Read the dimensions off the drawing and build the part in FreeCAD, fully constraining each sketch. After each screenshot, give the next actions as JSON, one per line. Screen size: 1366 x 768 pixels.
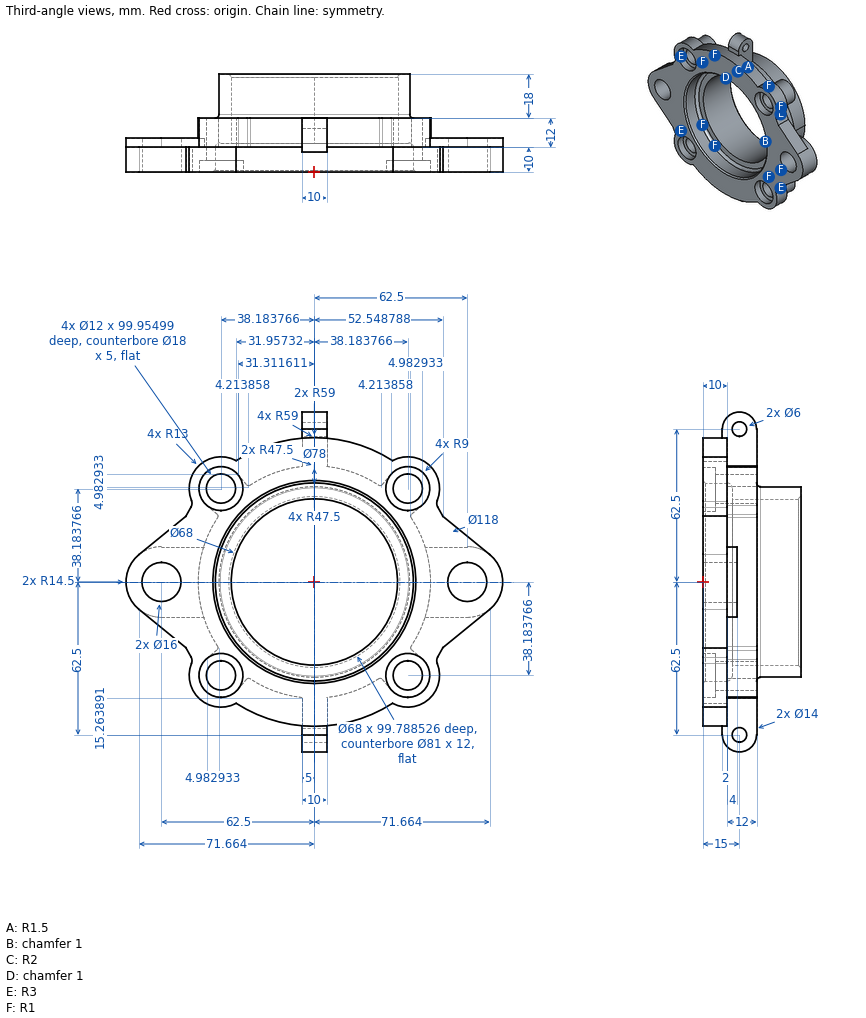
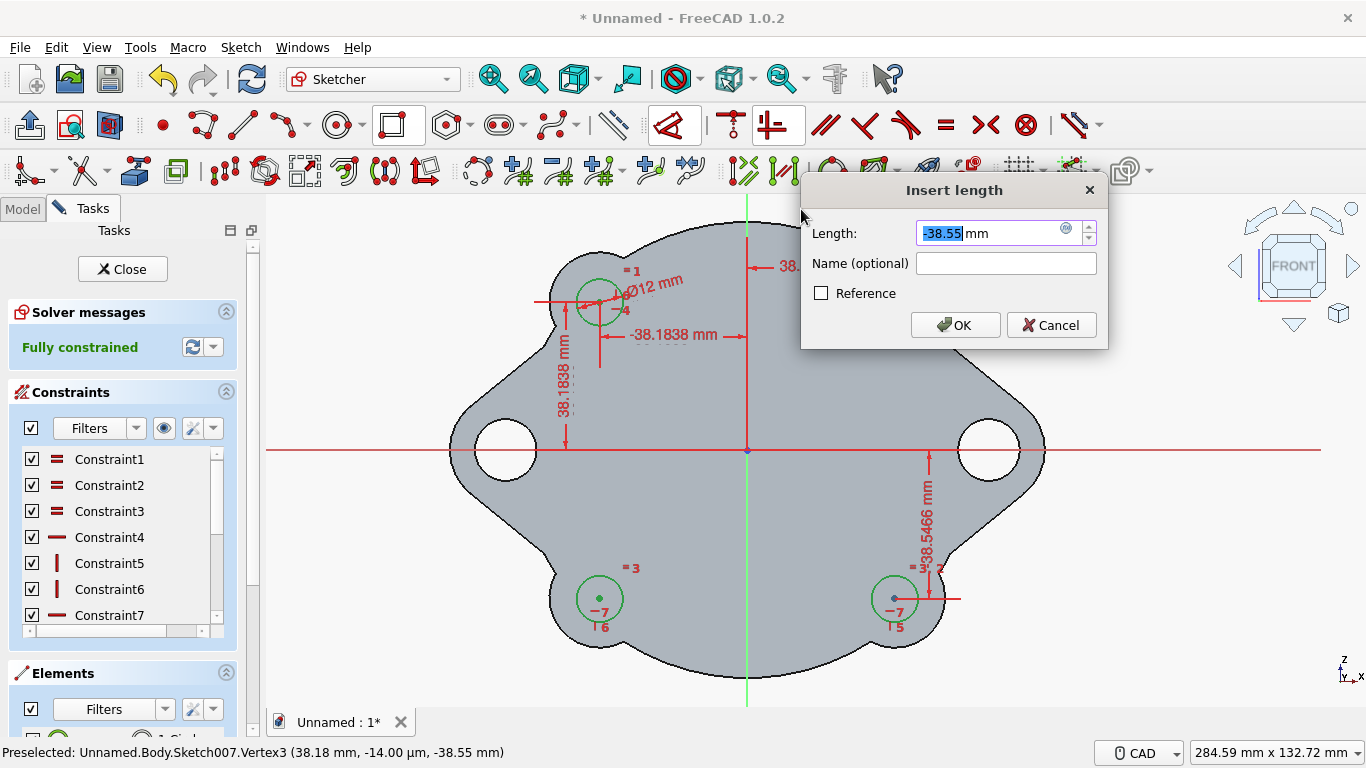
{"action": "type", "text": "-38.183766"}
{"action": "key", "text": "Return"}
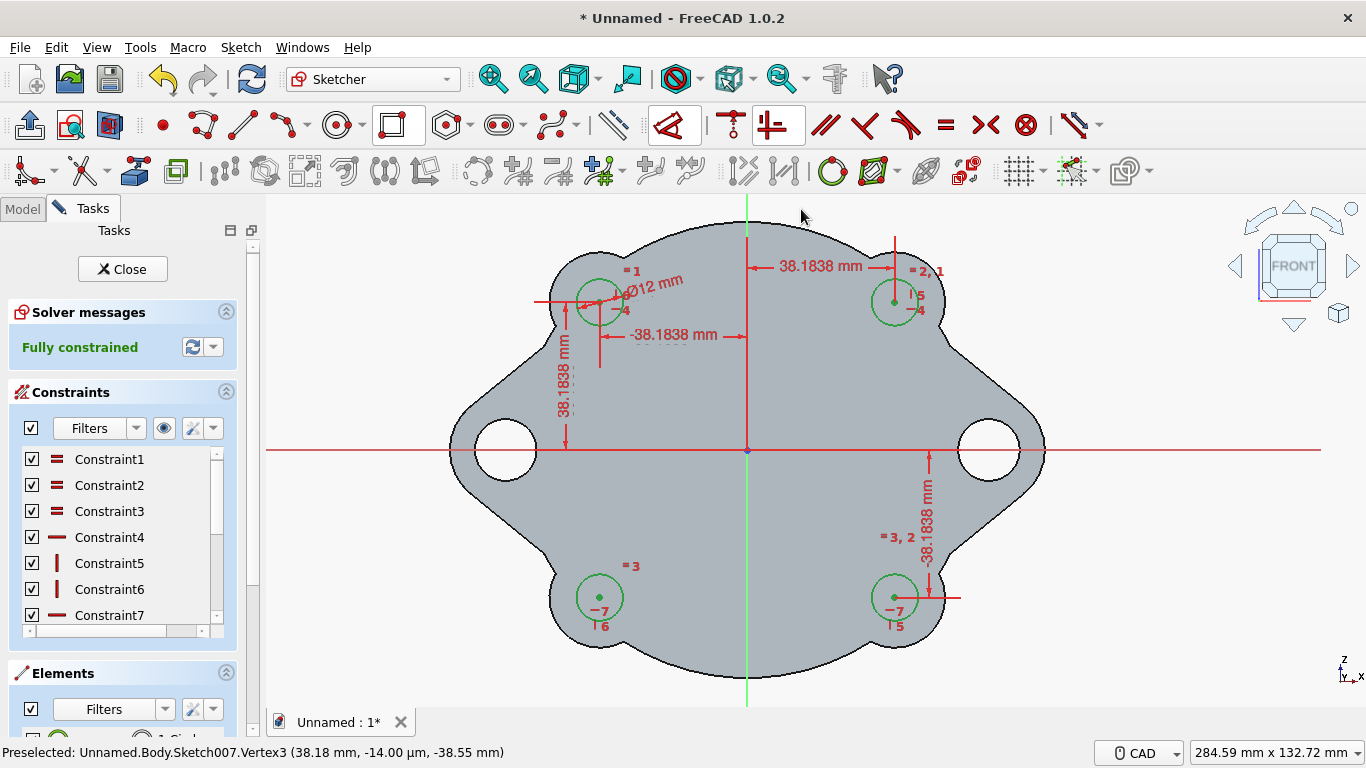
{"action": "left_click", "coordinate": [123, 269]}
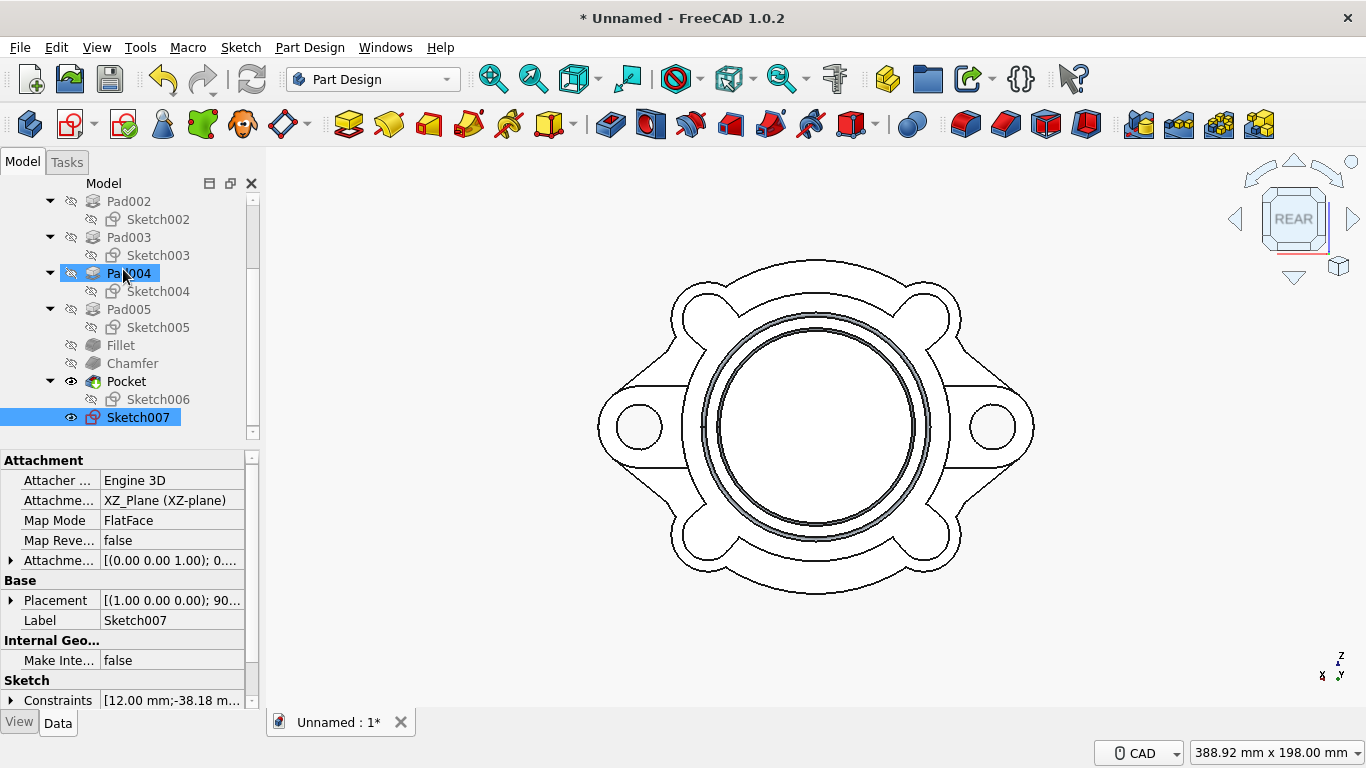
{"action": "left_click", "coordinate": [652, 124]}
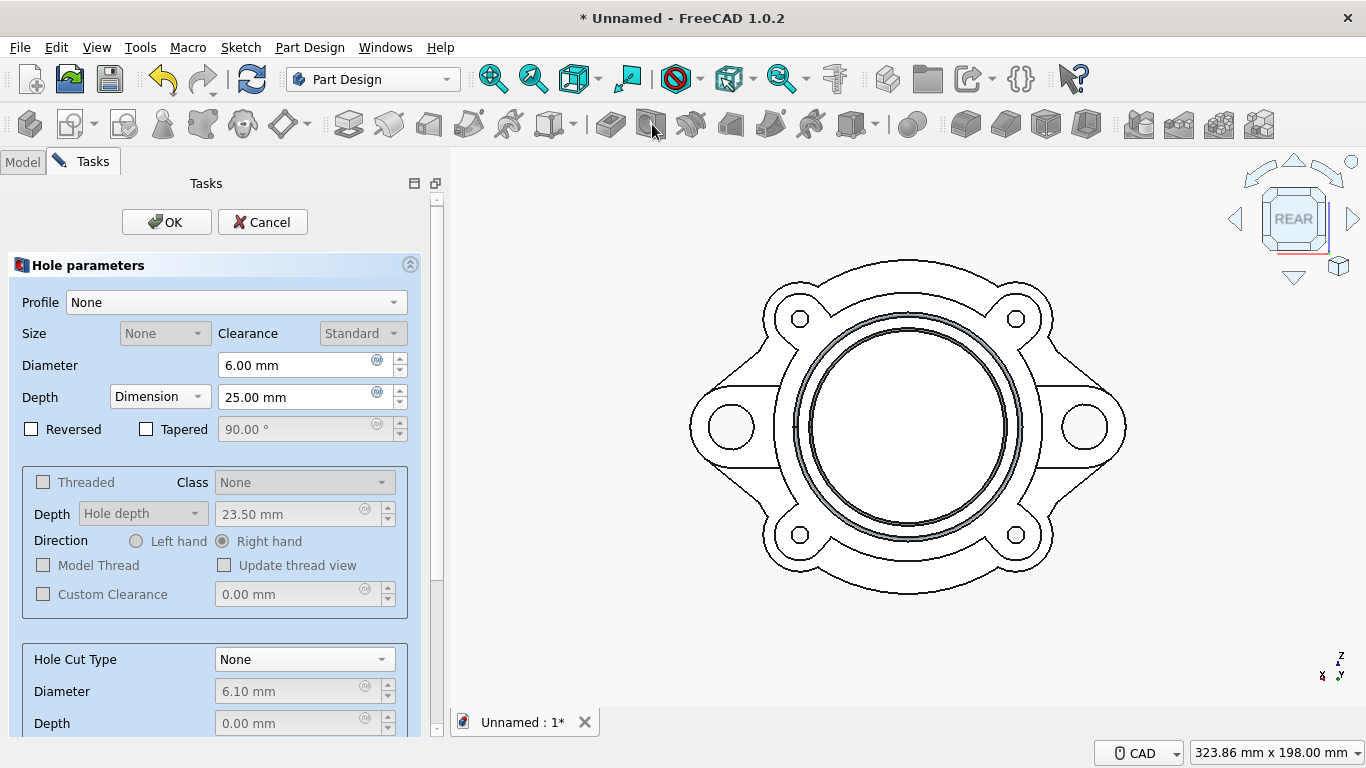
{"action": "triple_click", "coordinate": [305, 365]}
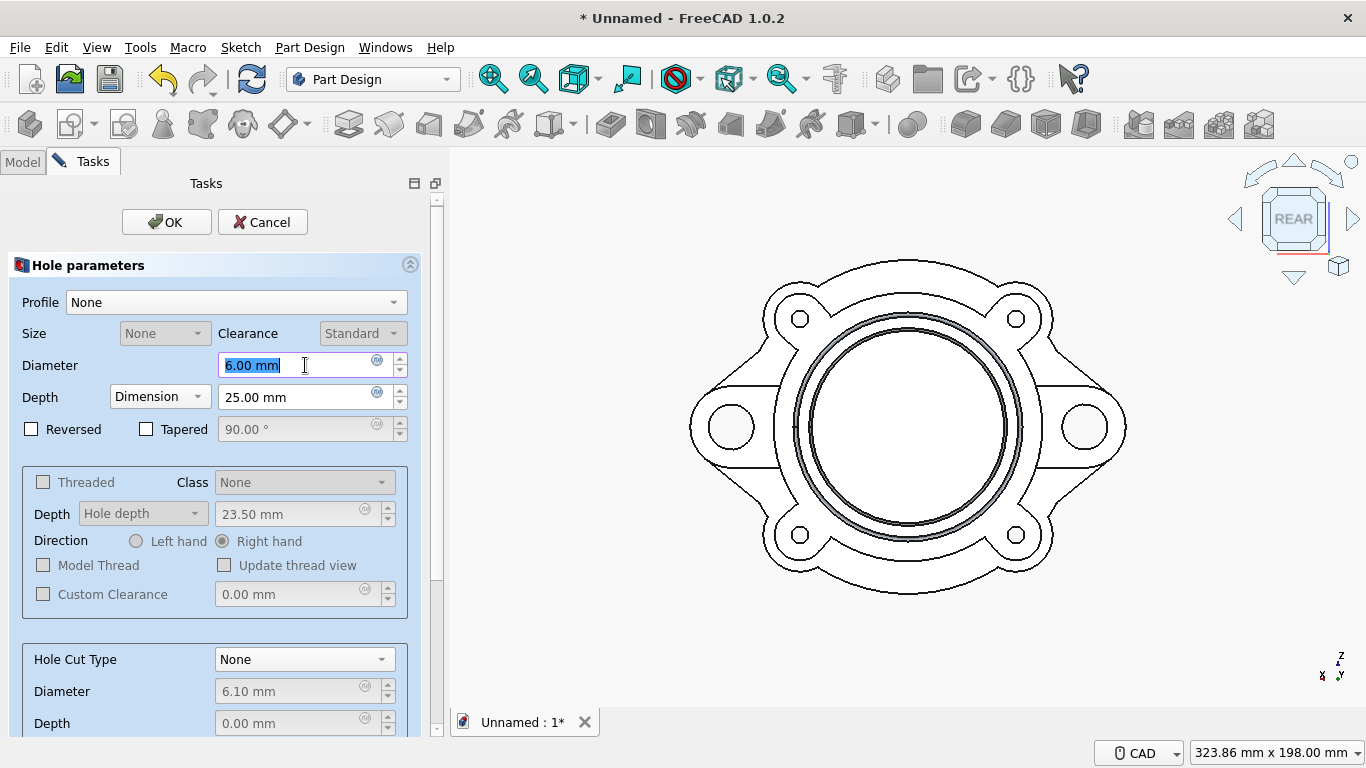
{"action": "type", "text": "12"}
{"action": "key", "text": "Tab"}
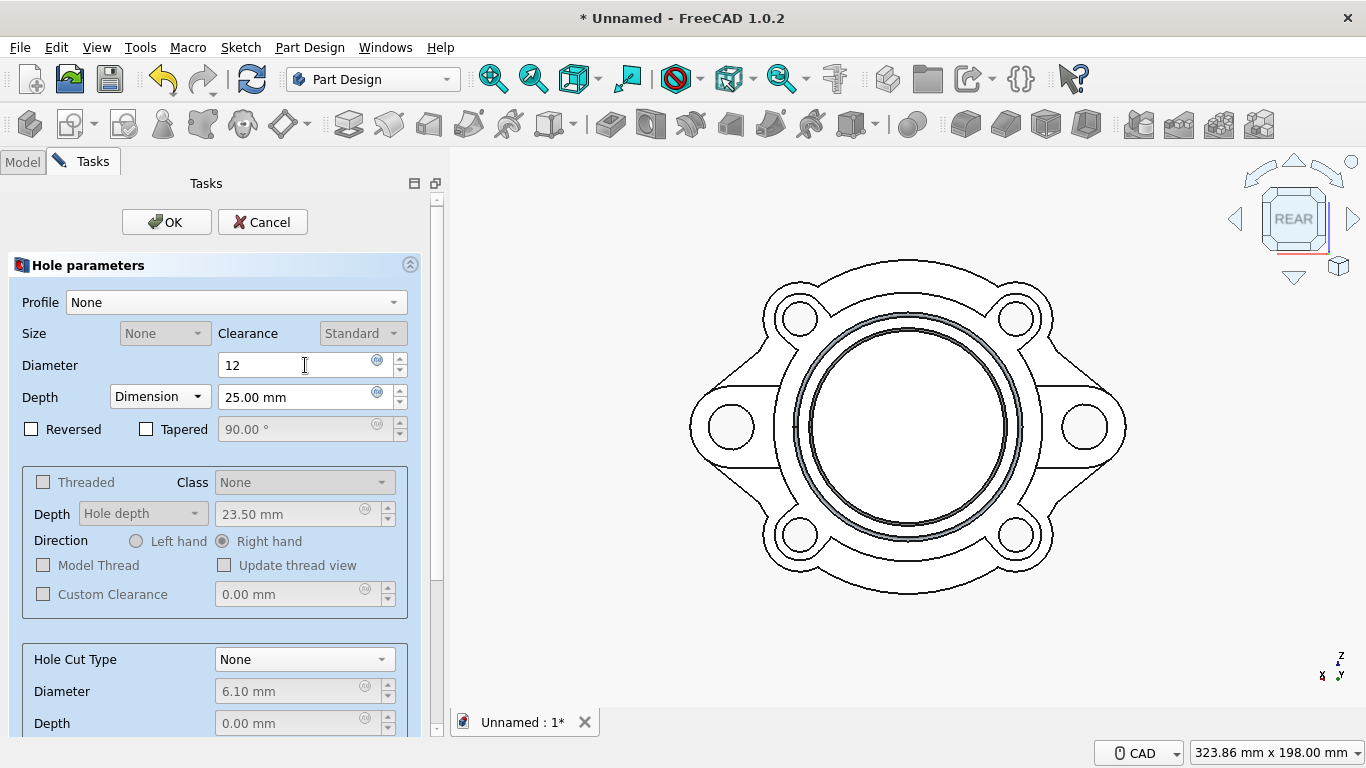
{"action": "triple_click", "coordinate": [305, 397]}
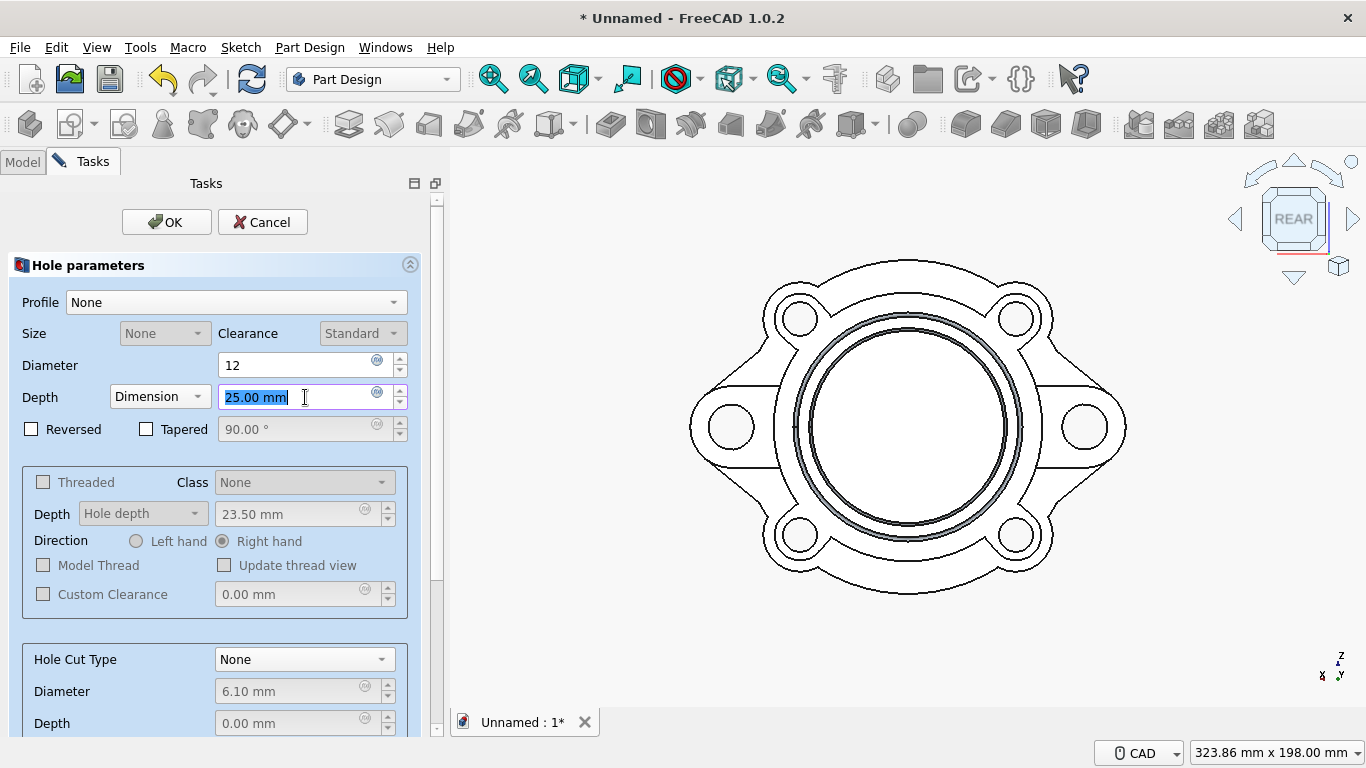
{"action": "type", "text": "99.95499"}
{"action": "key", "text": "Tab"}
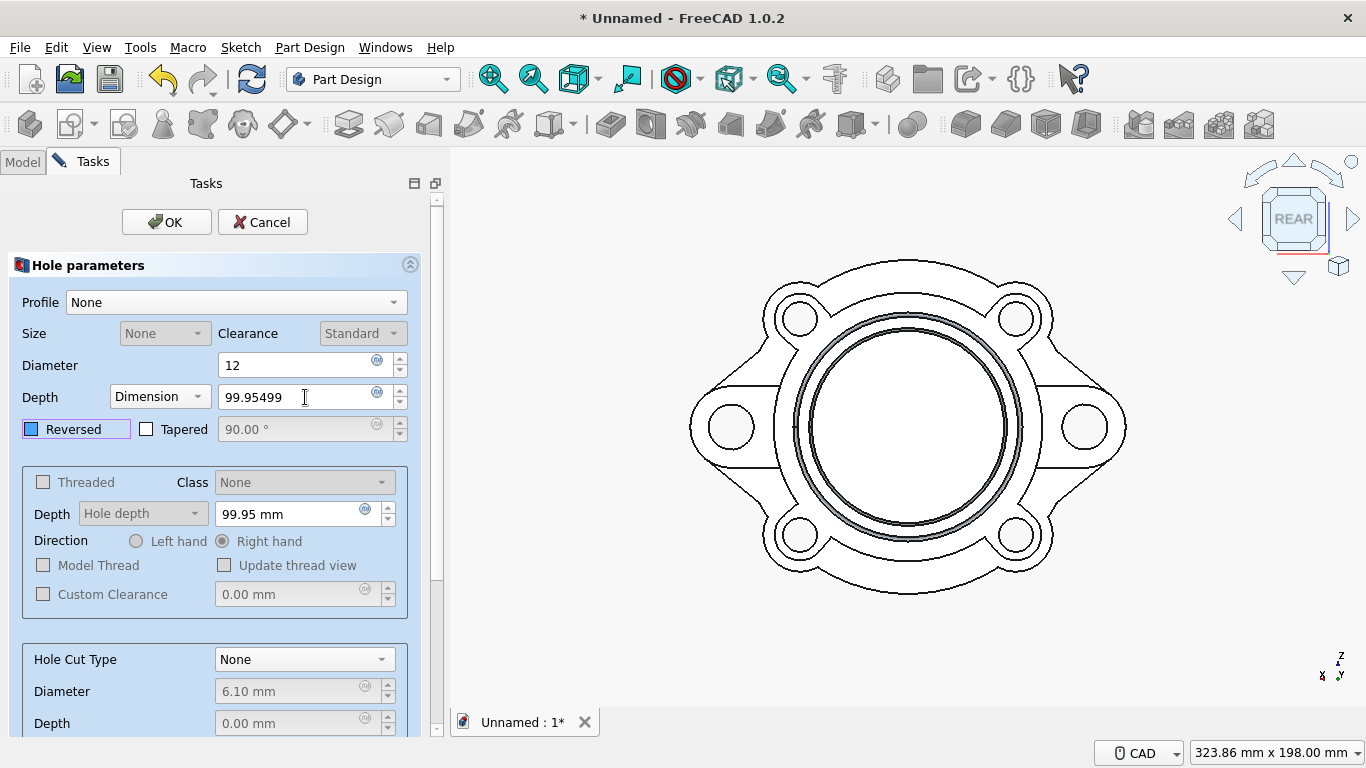
{"action": "left_click", "coordinate": [306, 660]}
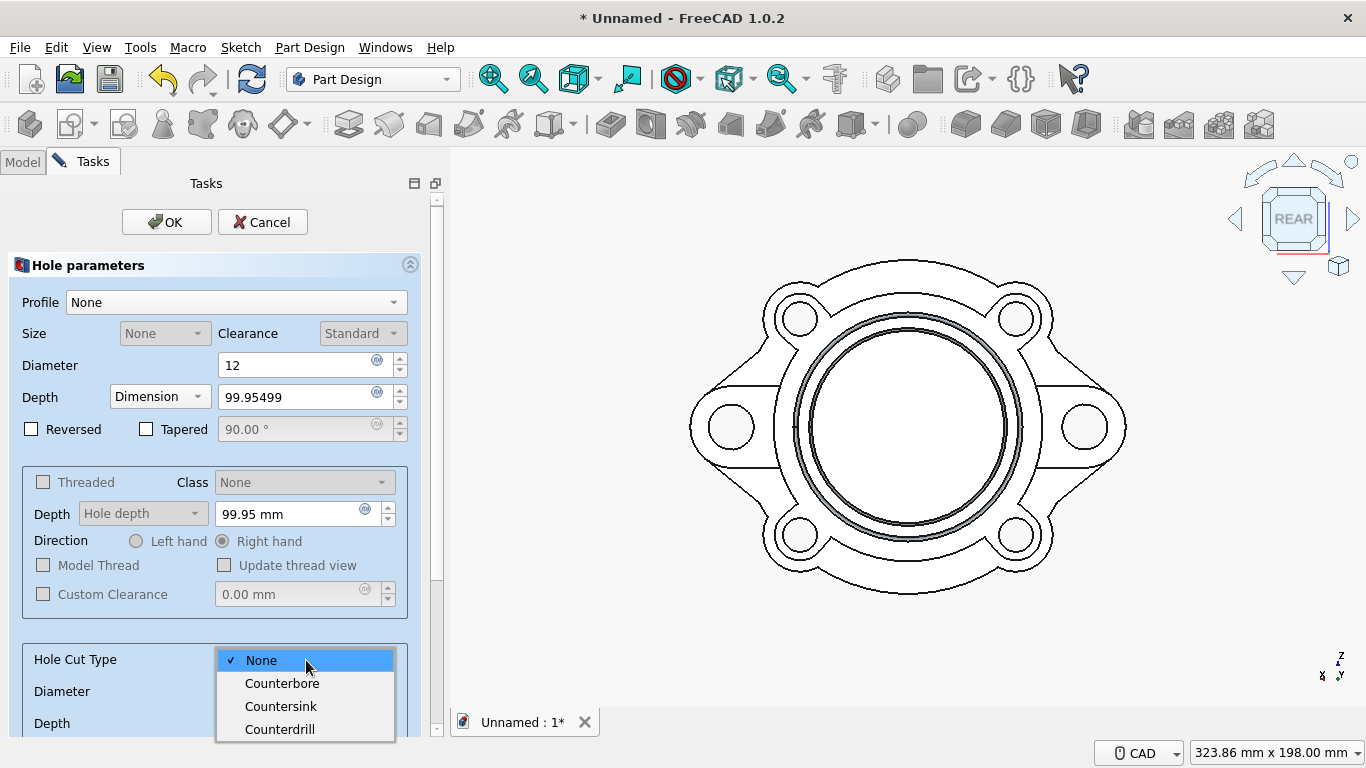
{"action": "left_click", "coordinate": [304, 684]}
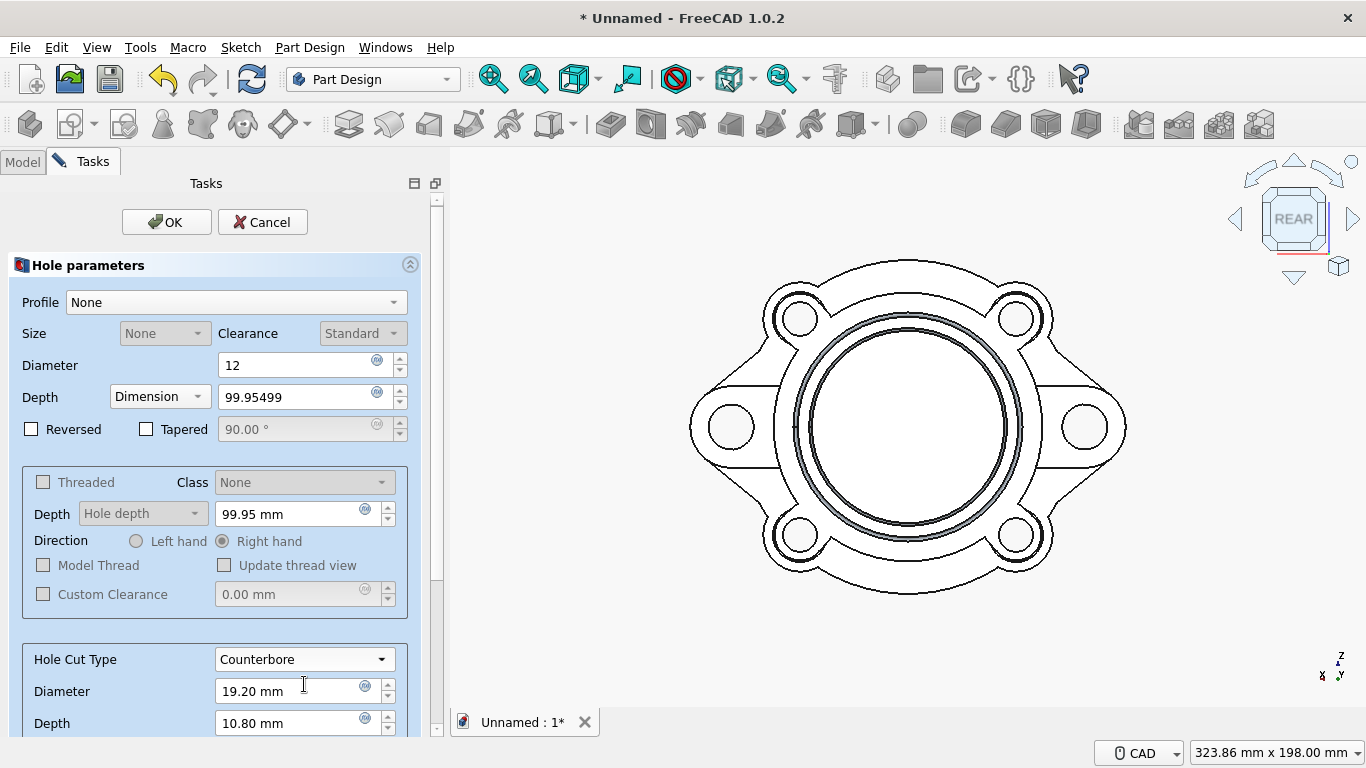
{"action": "triple_click", "coordinate": [298, 691]}